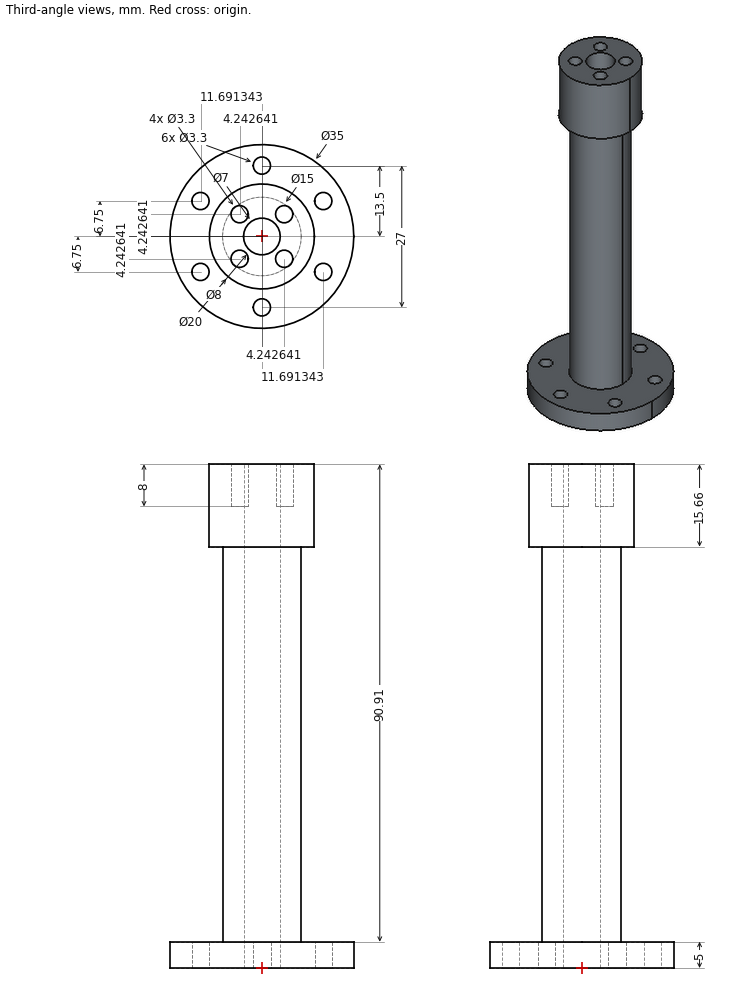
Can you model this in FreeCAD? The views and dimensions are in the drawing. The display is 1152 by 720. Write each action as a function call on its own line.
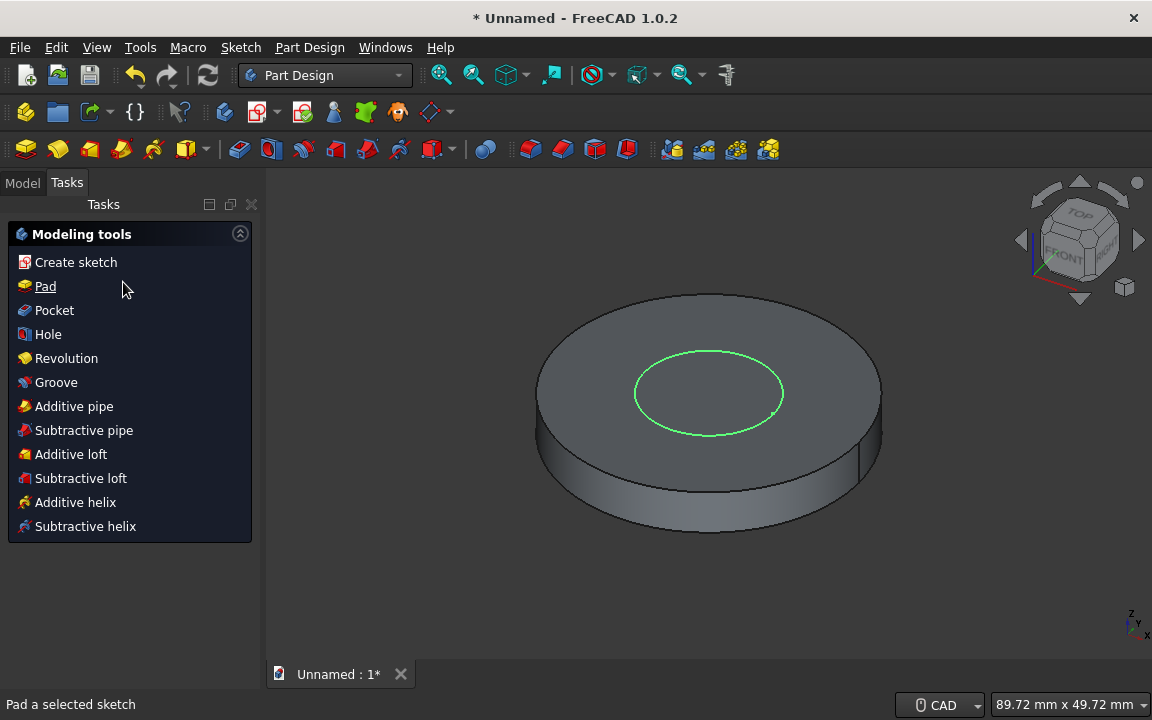
click(26, 150)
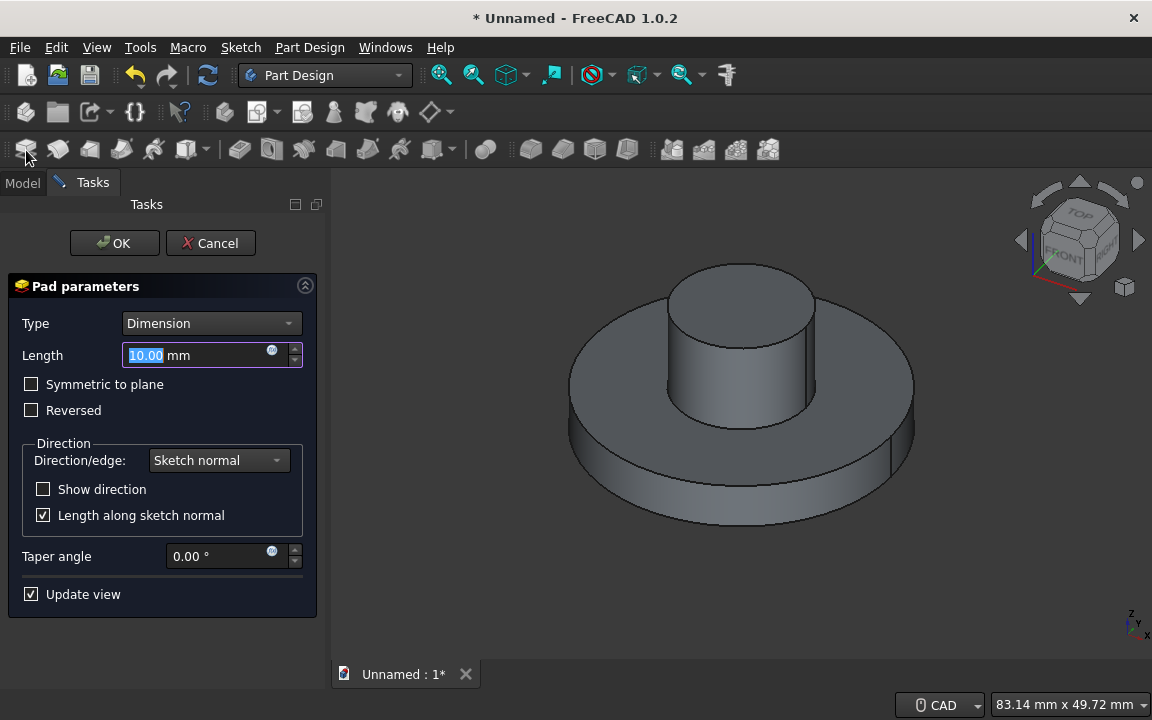
text(90.91)
key(Tab)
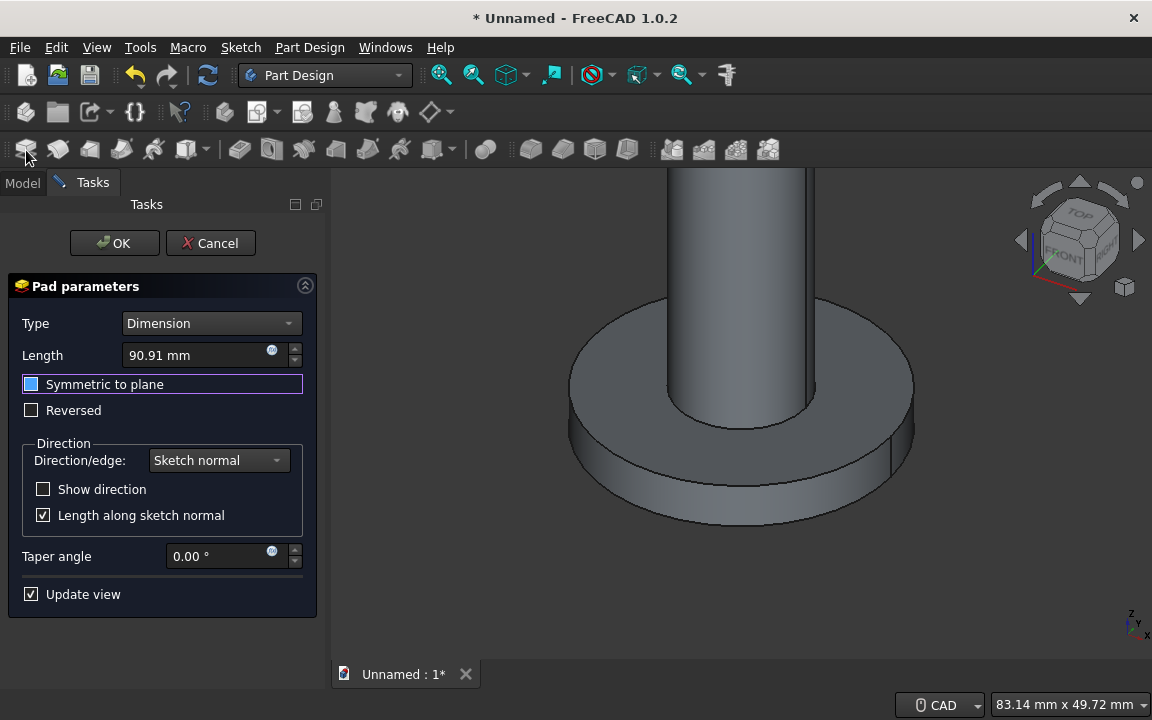
click(115, 243)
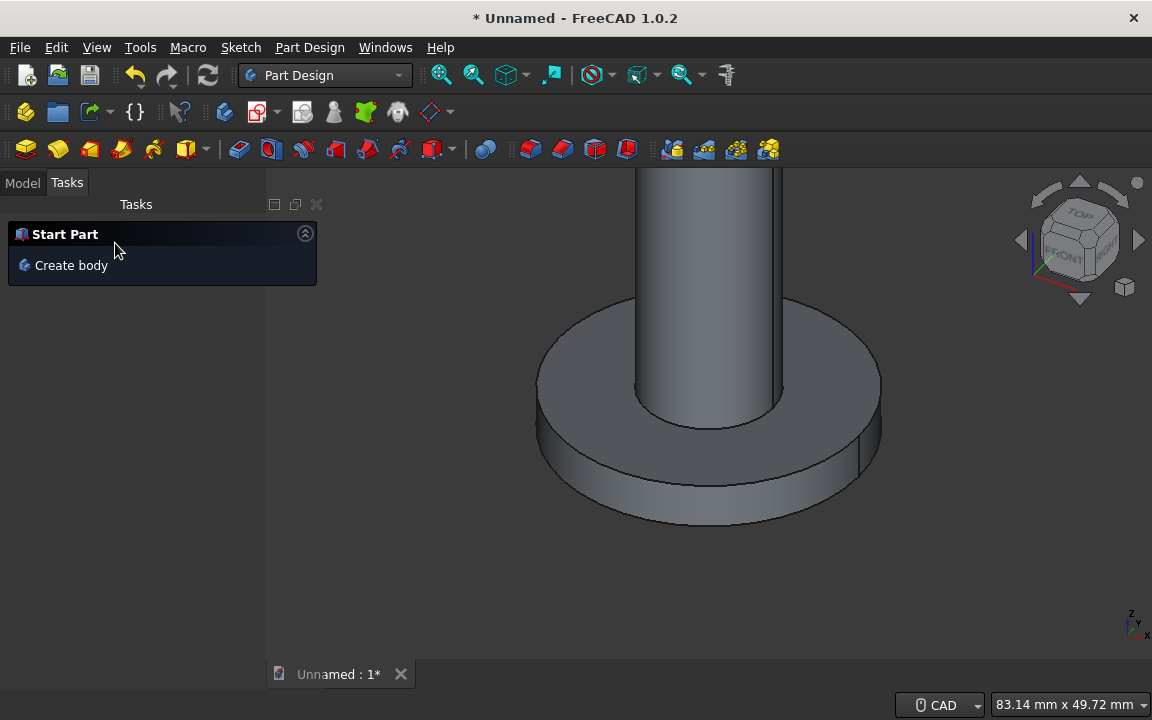
click(442, 76)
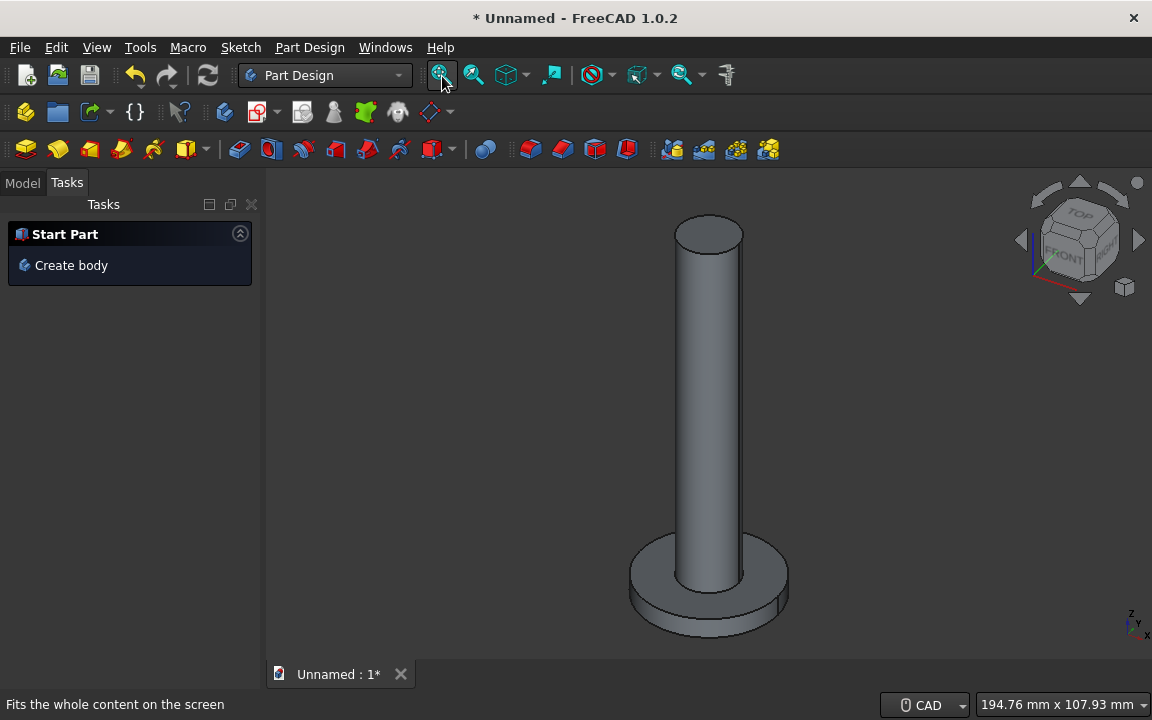
click(258, 112)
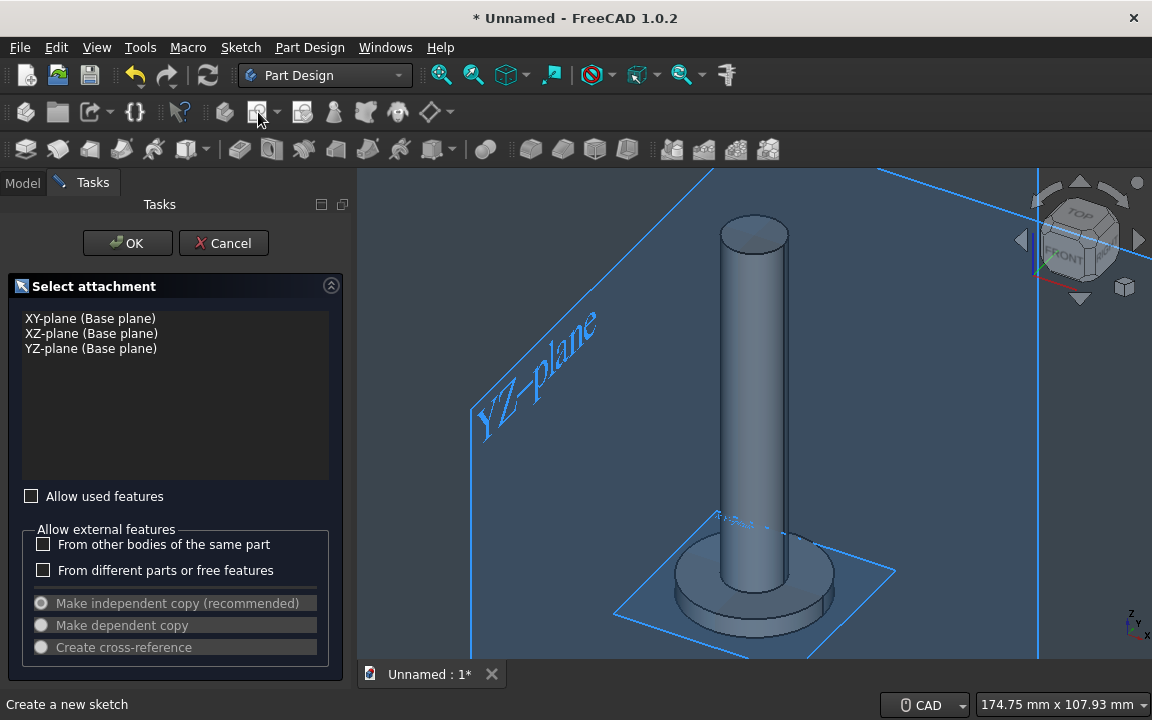
click(82, 318)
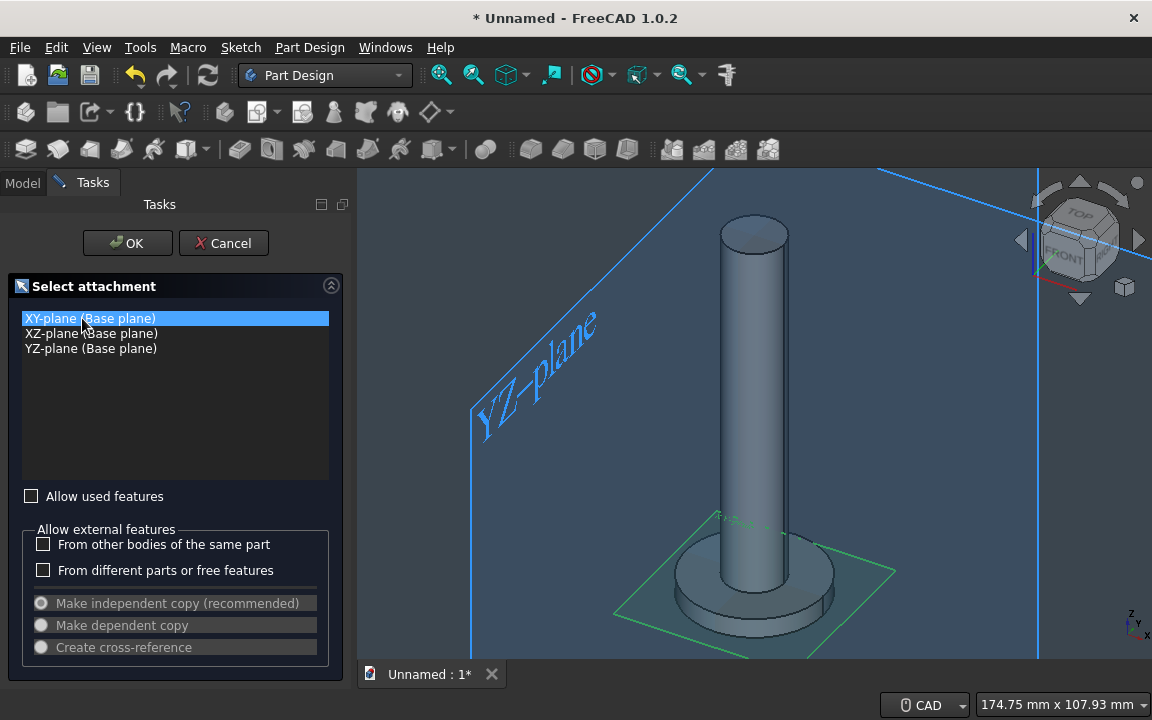
click(128, 243)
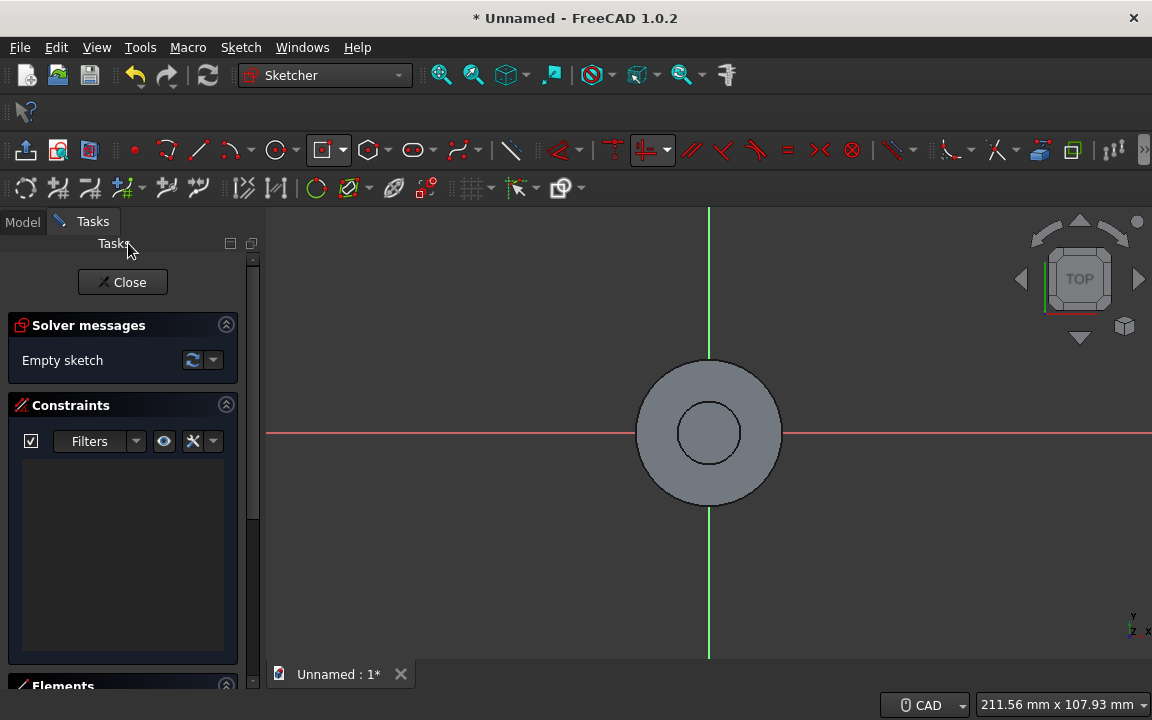
key(q)
key(s)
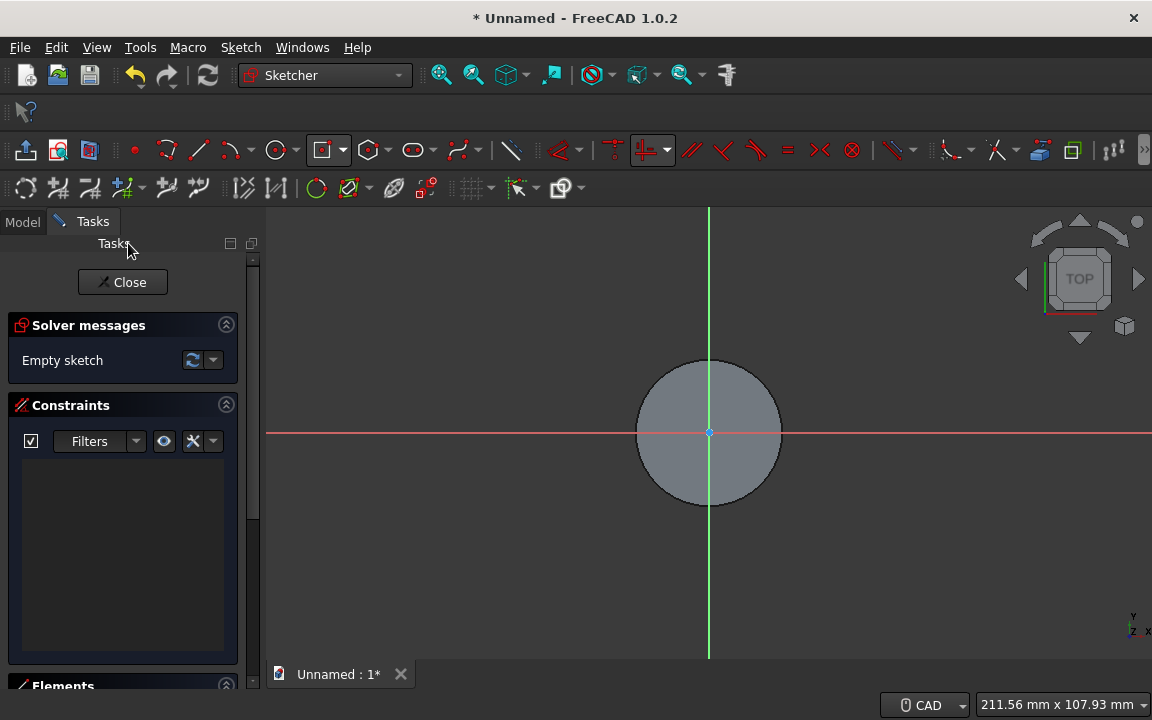
scroll(765, 433, up, 4)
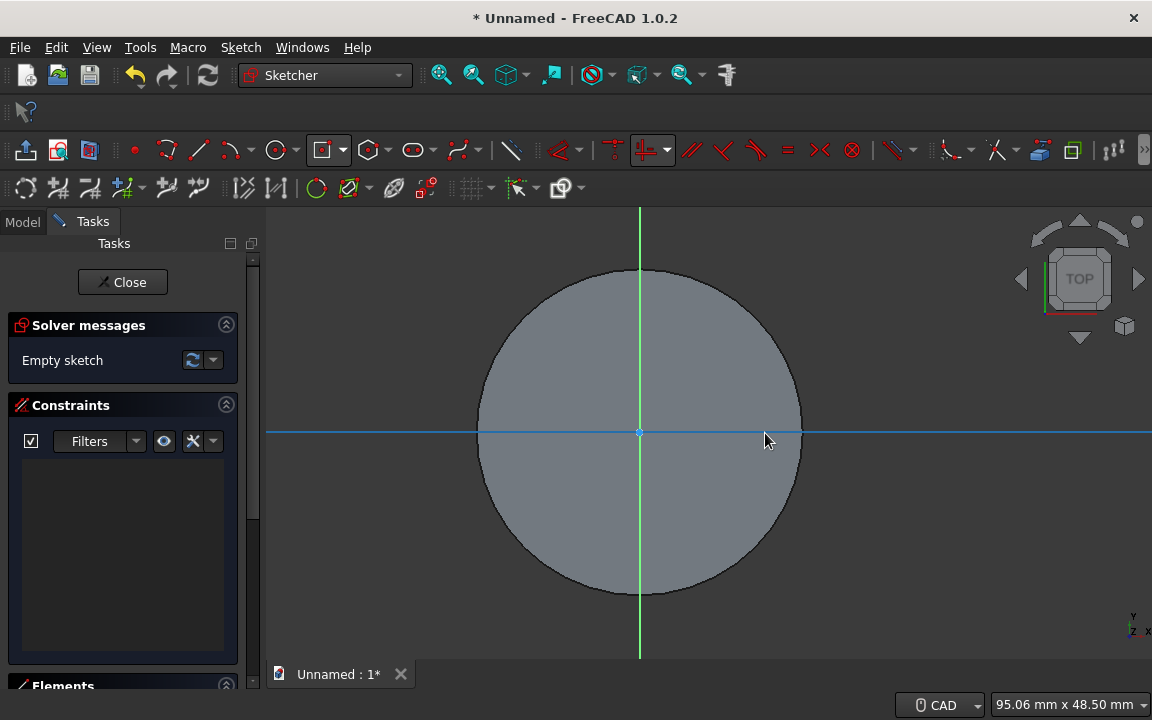
key(g)
key(c)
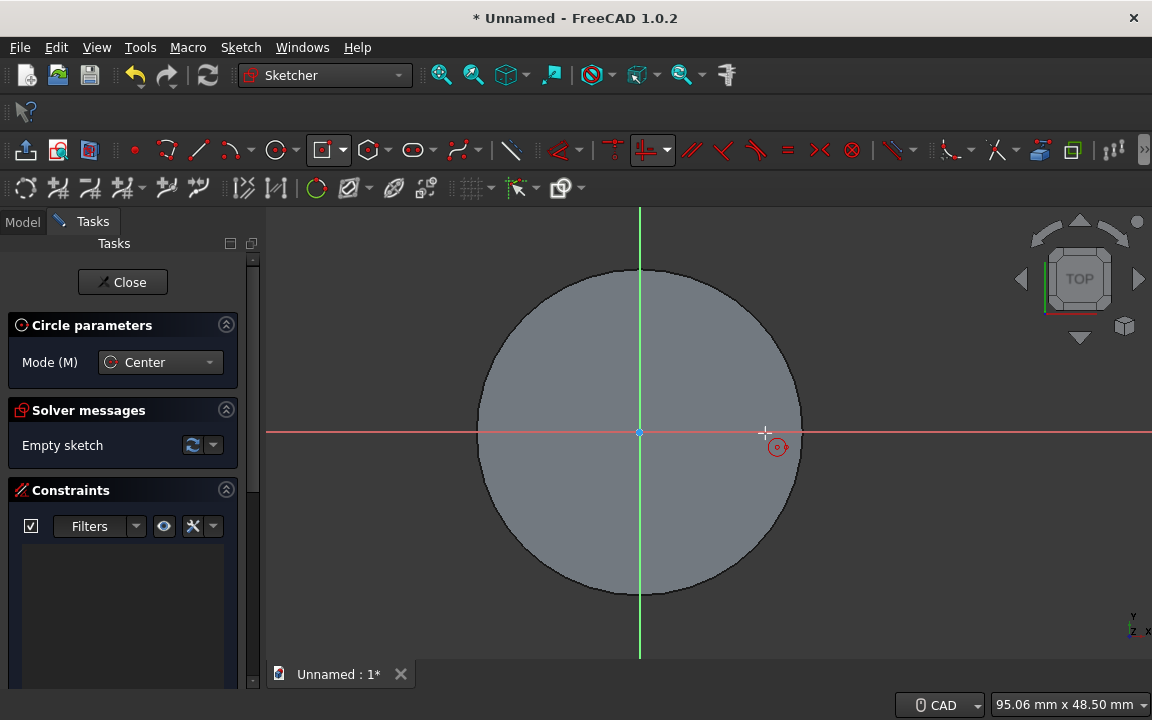
scroll(640, 307, up, 2)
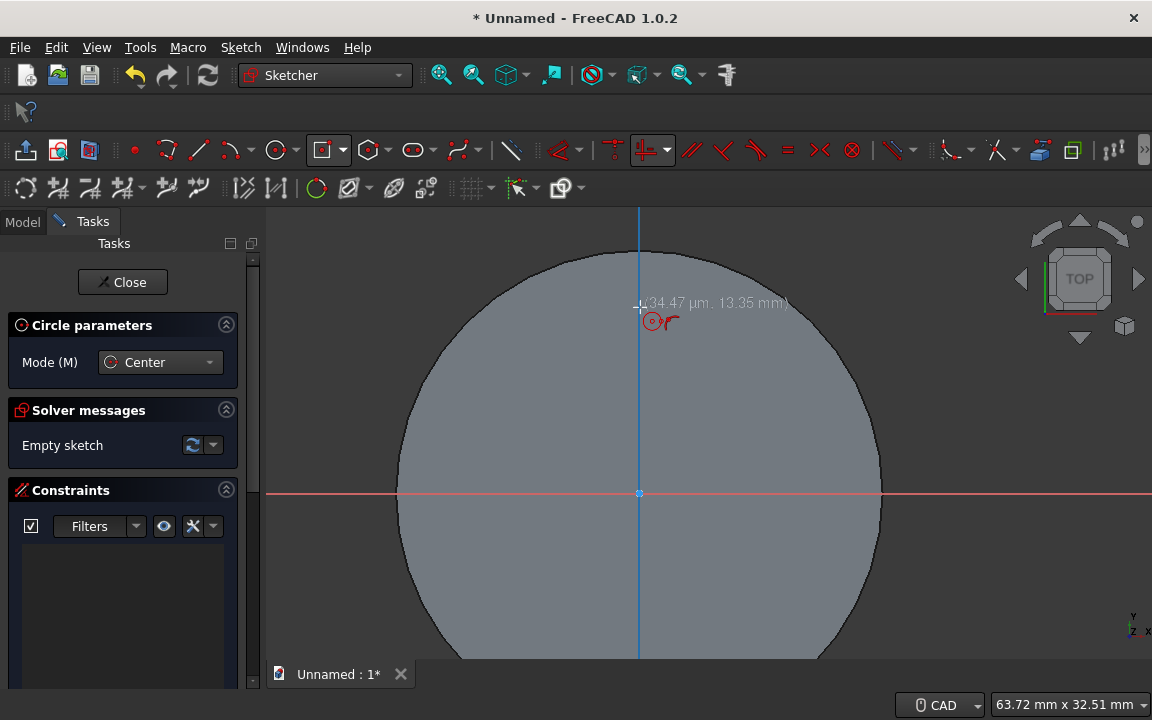
click(639, 306)
click(656, 290)